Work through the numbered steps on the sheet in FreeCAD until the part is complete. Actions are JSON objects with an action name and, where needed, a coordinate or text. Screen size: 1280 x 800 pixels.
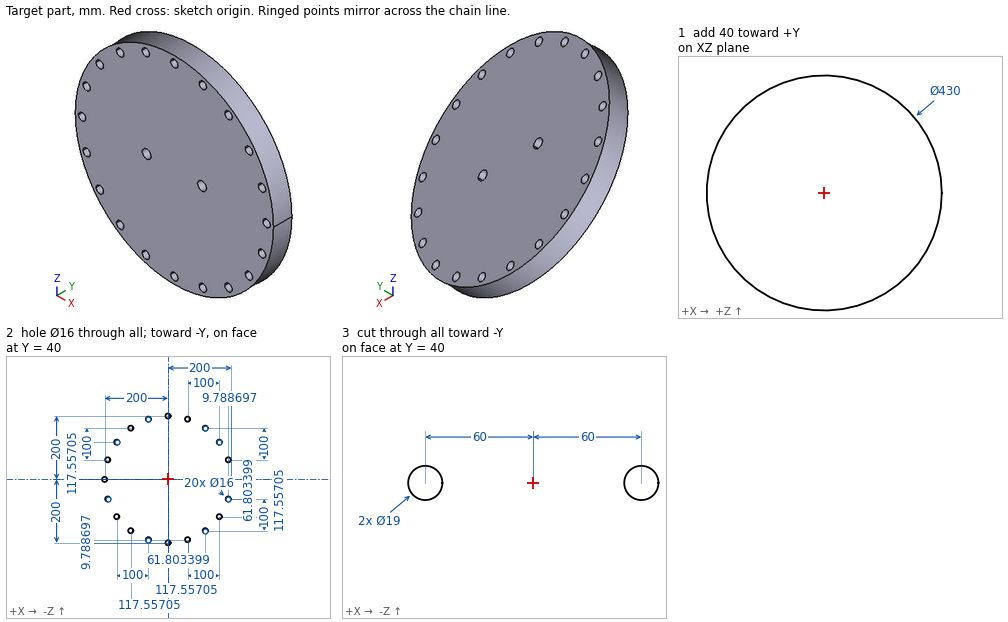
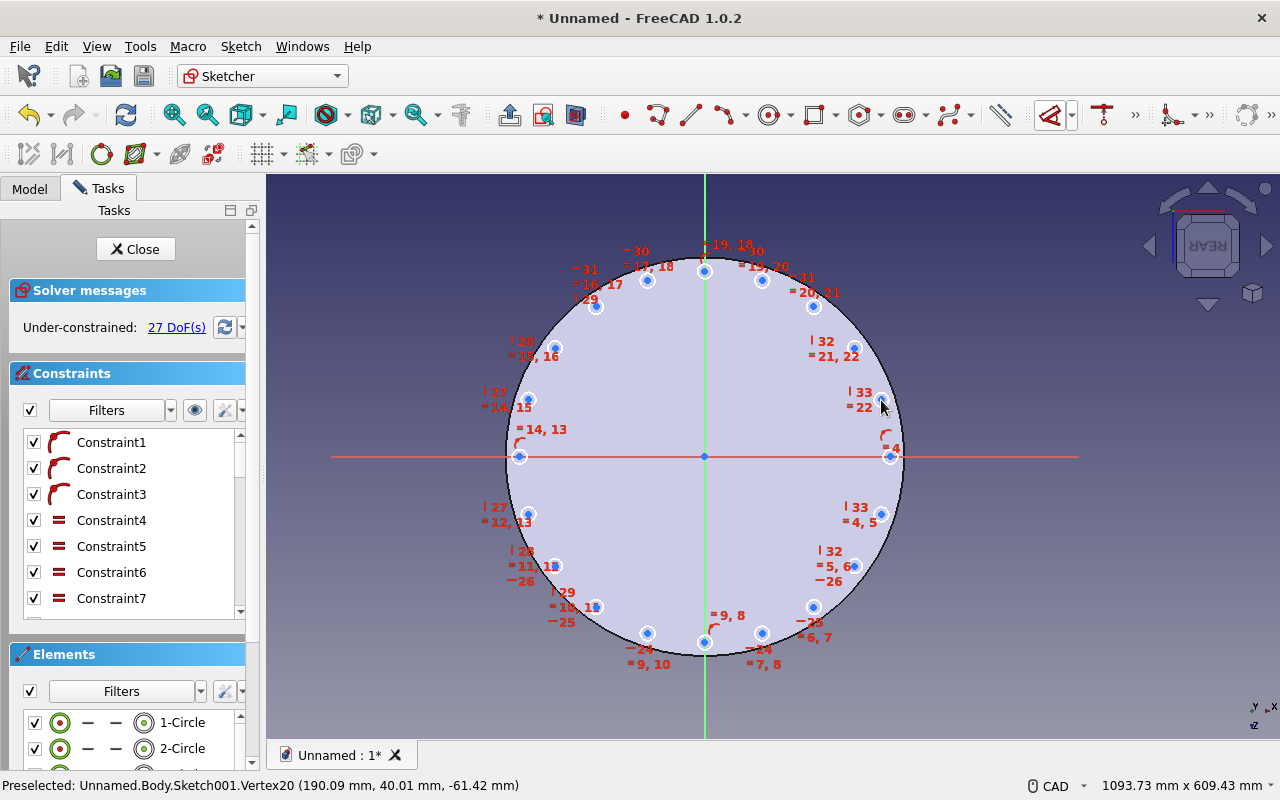
{"action": "left_click", "coordinate": [881, 514]}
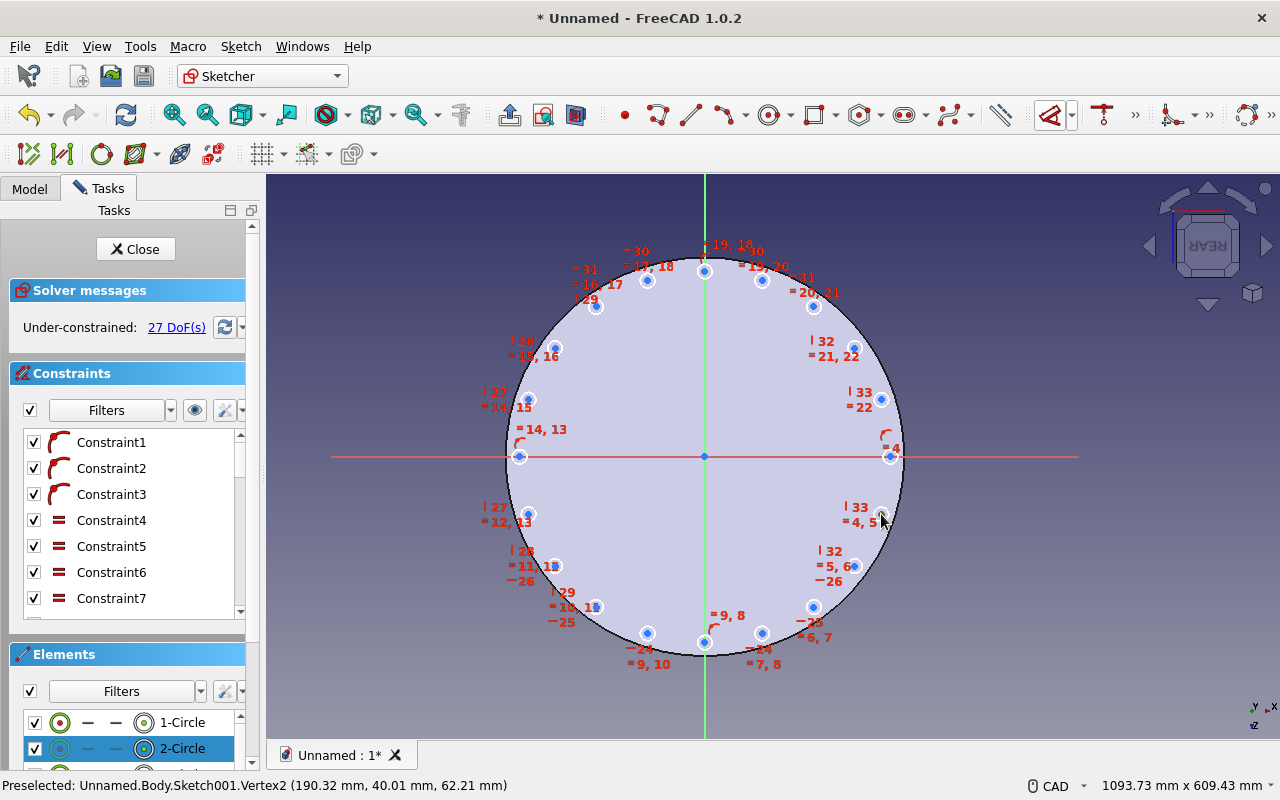
{"action": "left_click", "coordinate": [529, 514]}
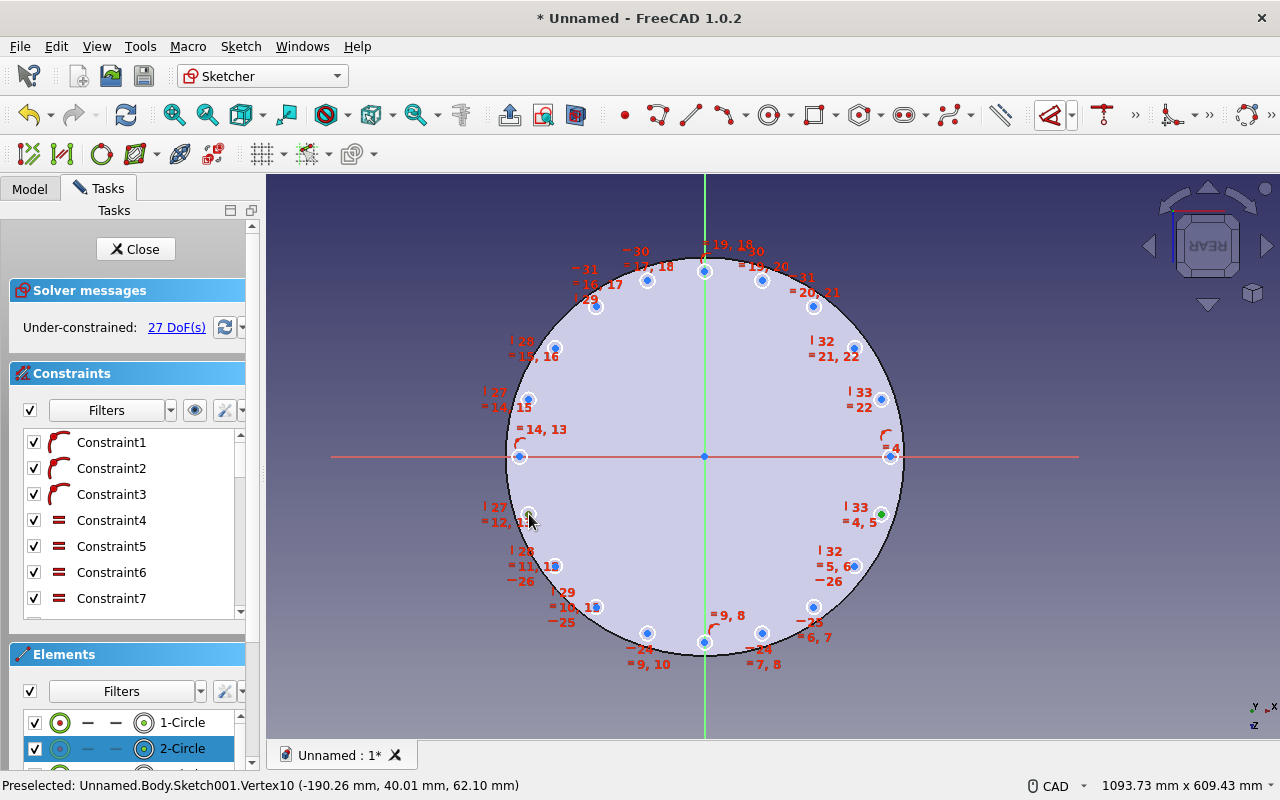
{"action": "left_click", "coordinate": [705, 602]}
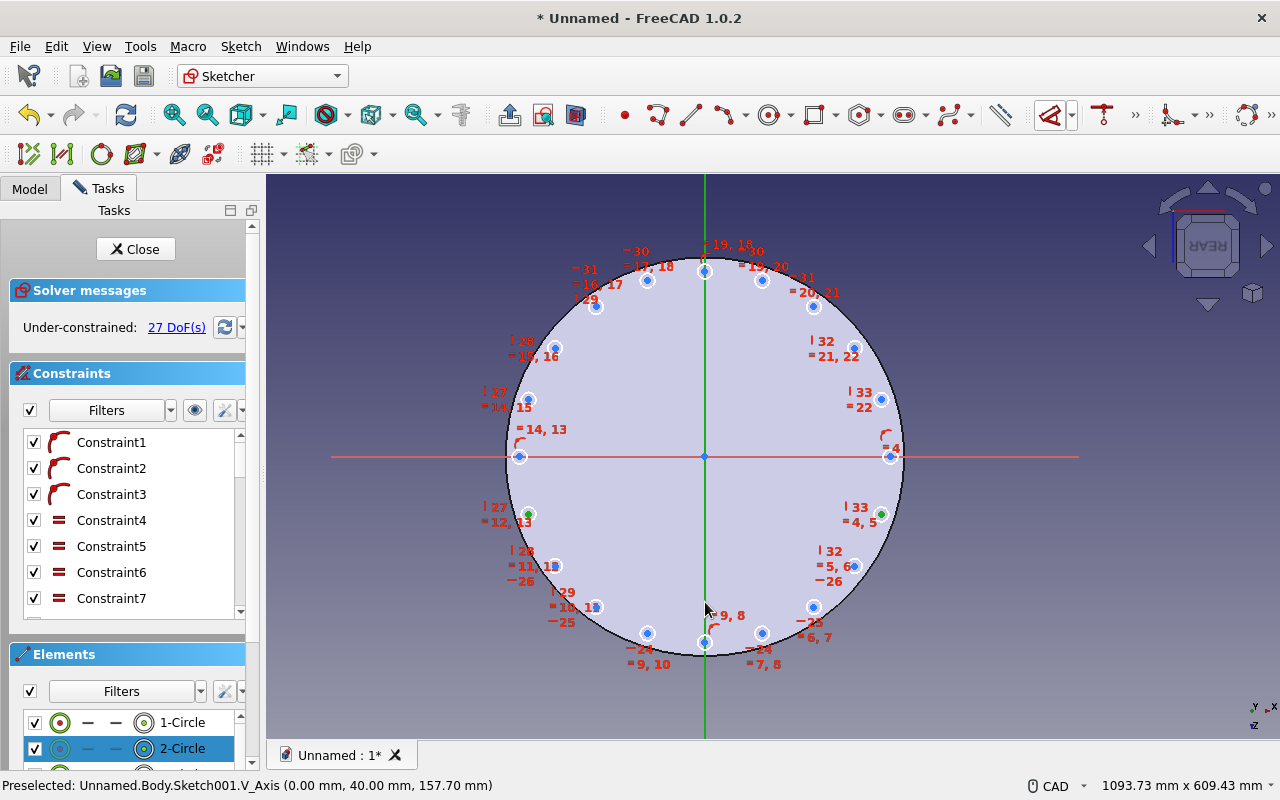
{"action": "key", "text": "s"}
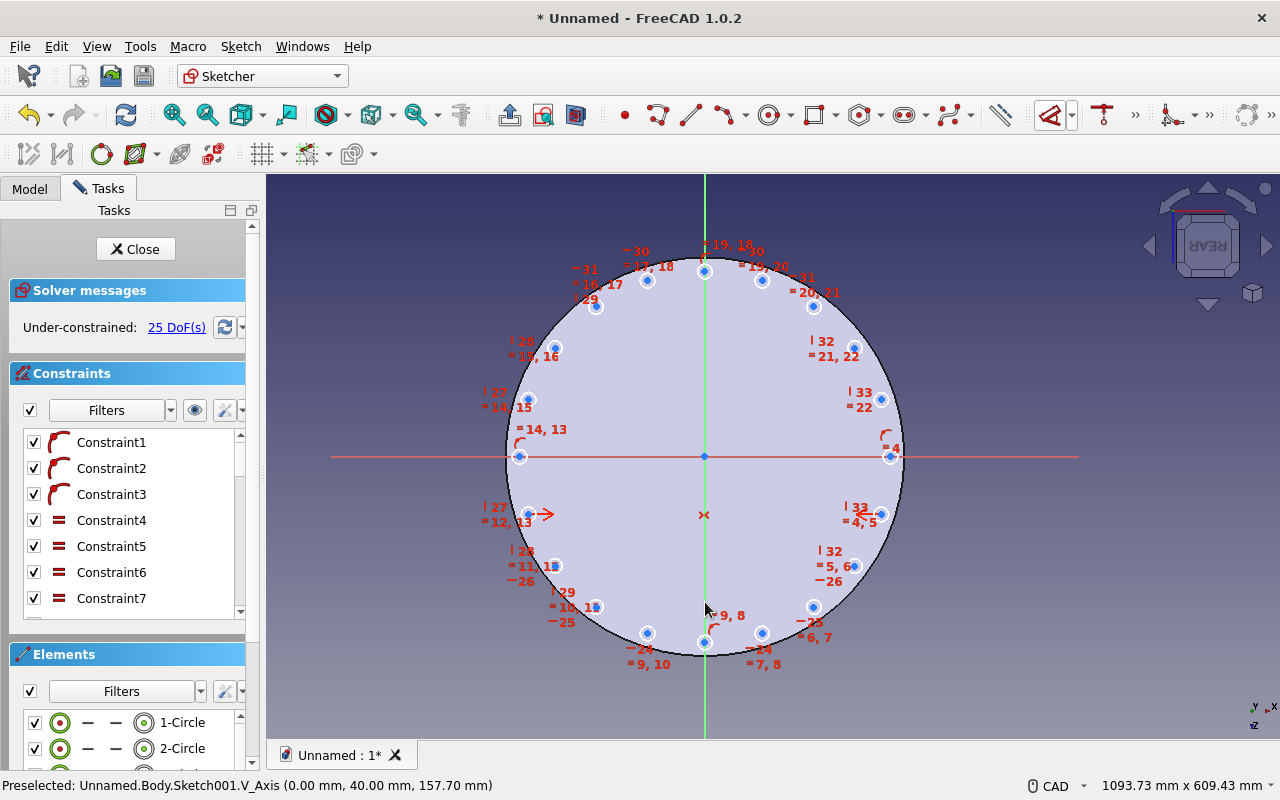
{"action": "left_click", "coordinate": [648, 634]}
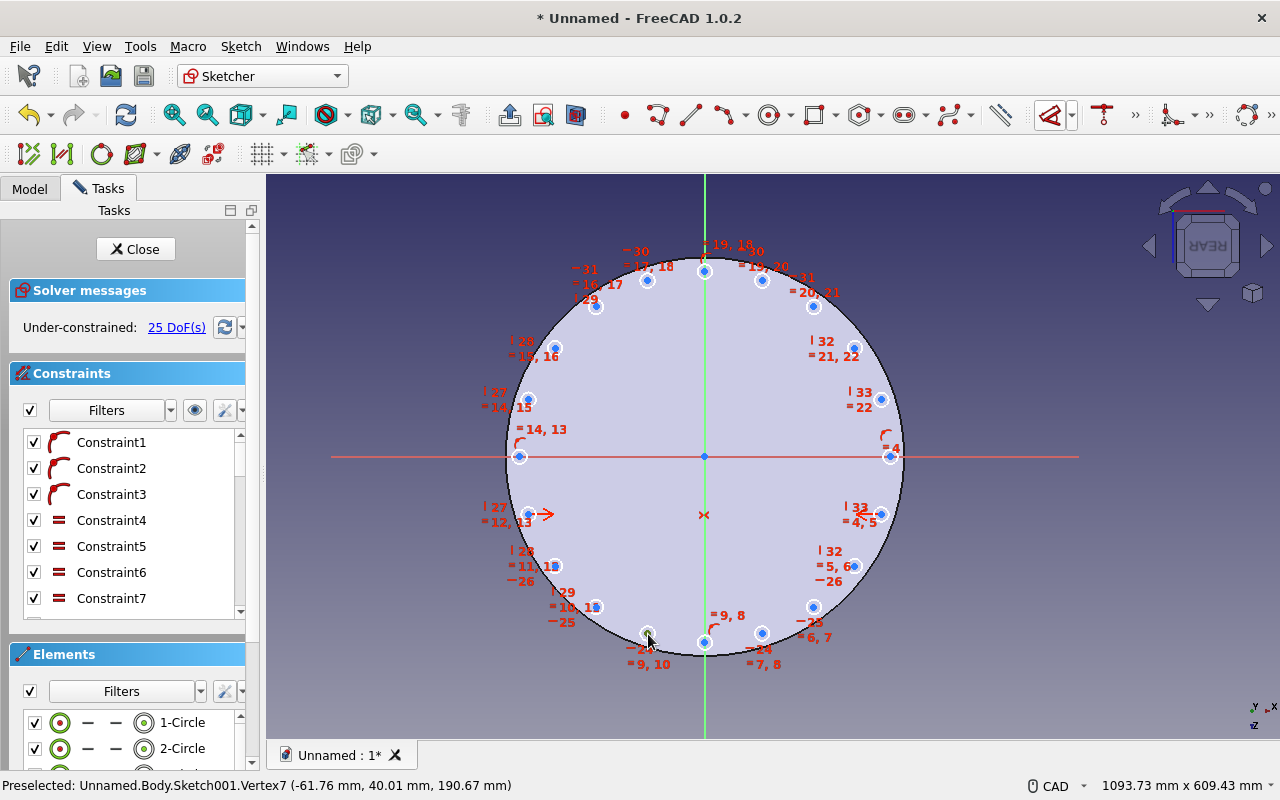
{"action": "left_click", "coordinate": [648, 281]}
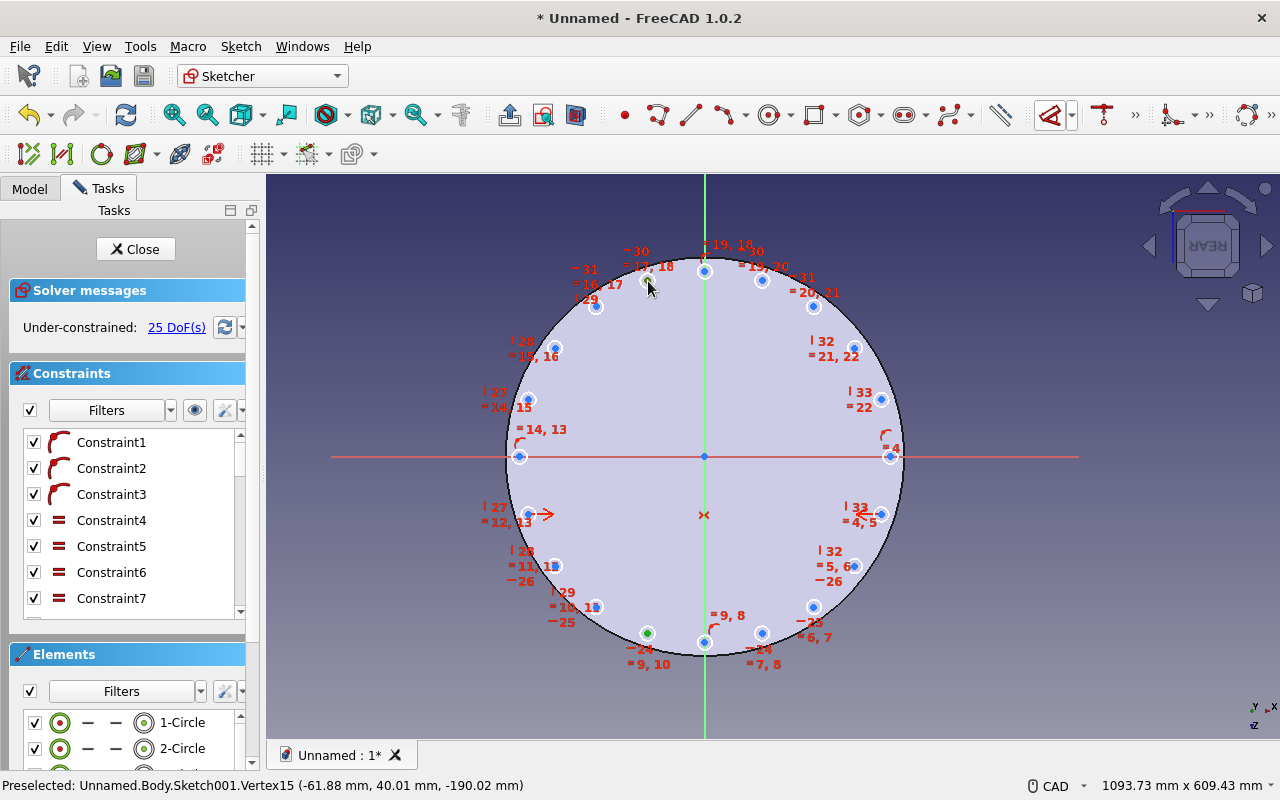
{"action": "left_click", "coordinate": [353, 457]}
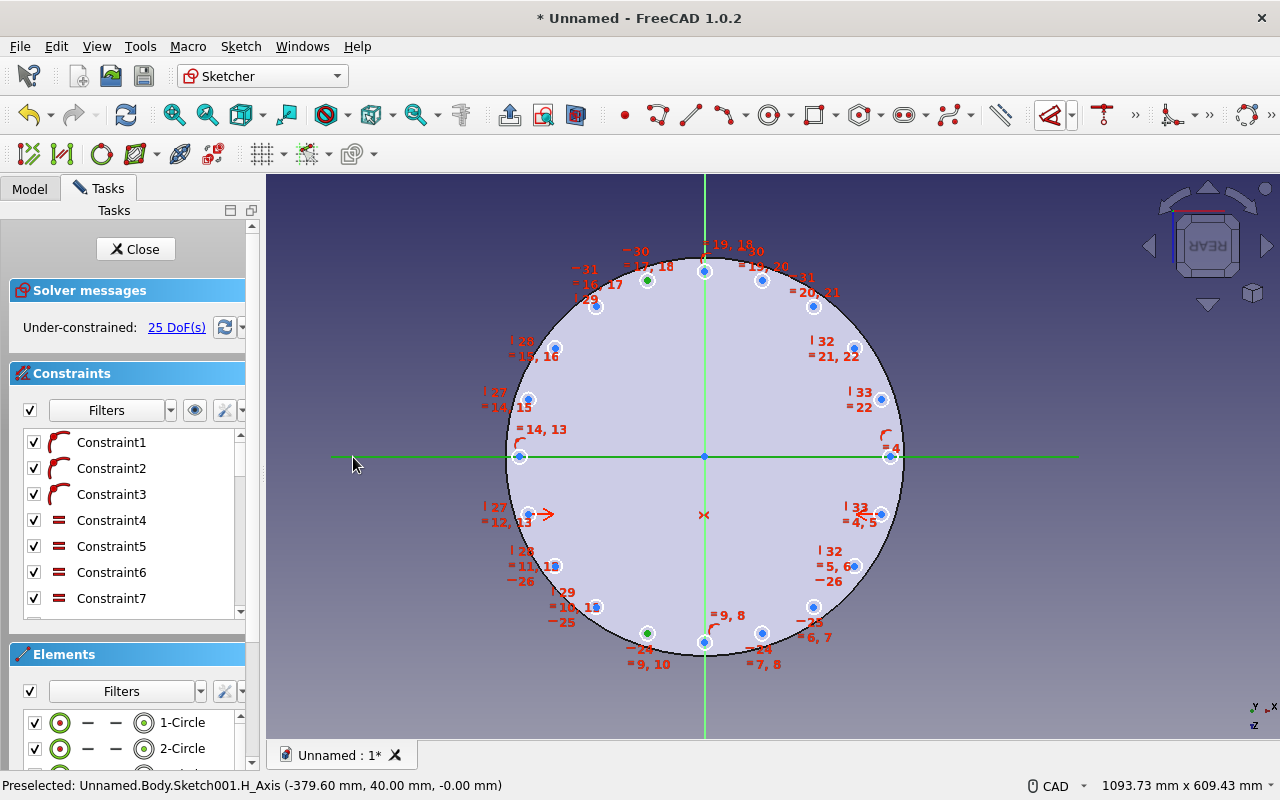
{"action": "key", "text": "s"}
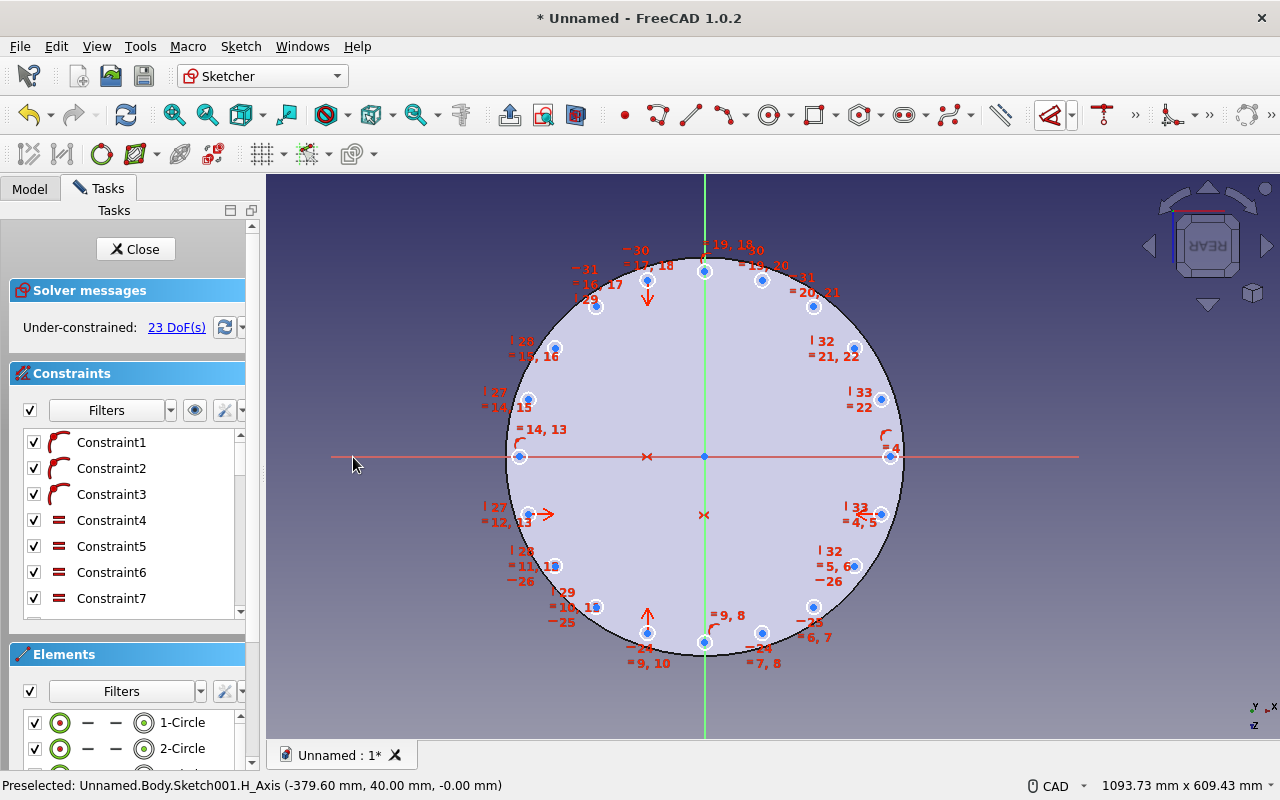
{"action": "left_click", "coordinate": [814, 607]}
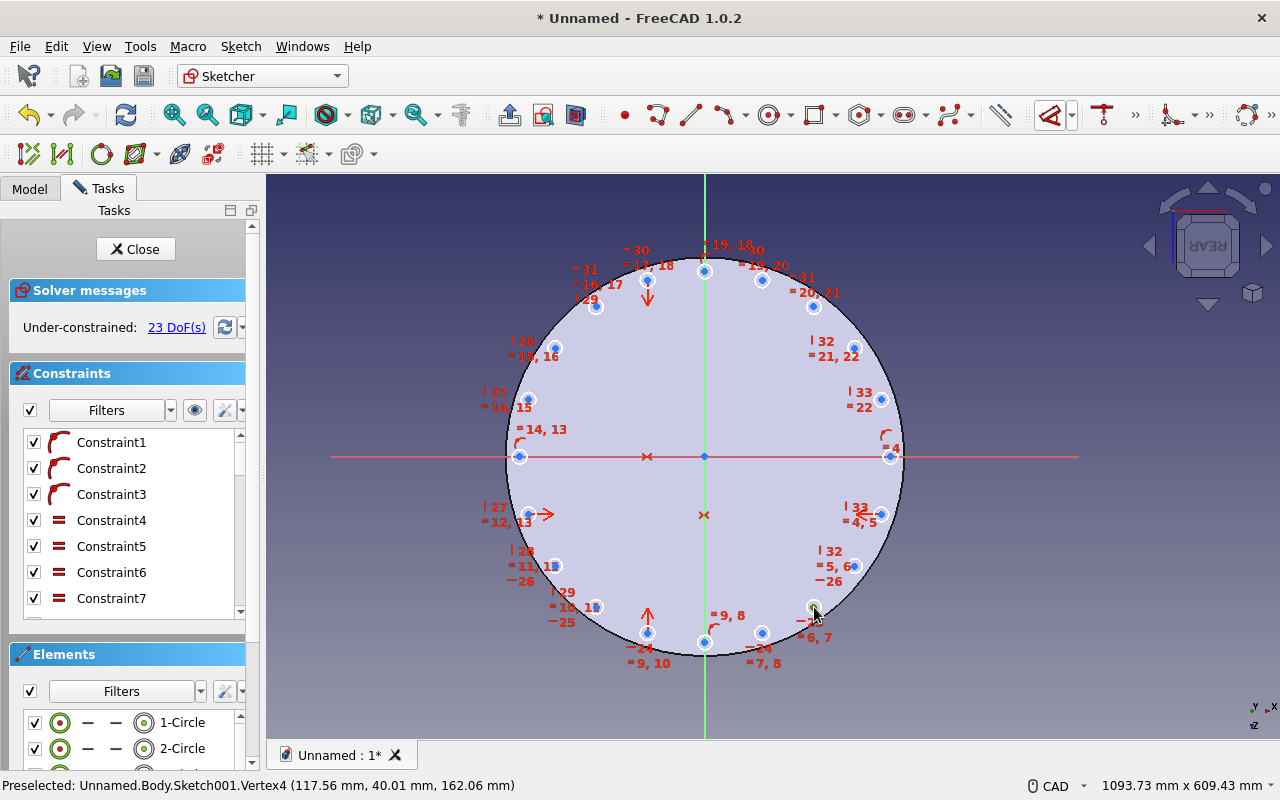
{"action": "left_click", "coordinate": [814, 307]}